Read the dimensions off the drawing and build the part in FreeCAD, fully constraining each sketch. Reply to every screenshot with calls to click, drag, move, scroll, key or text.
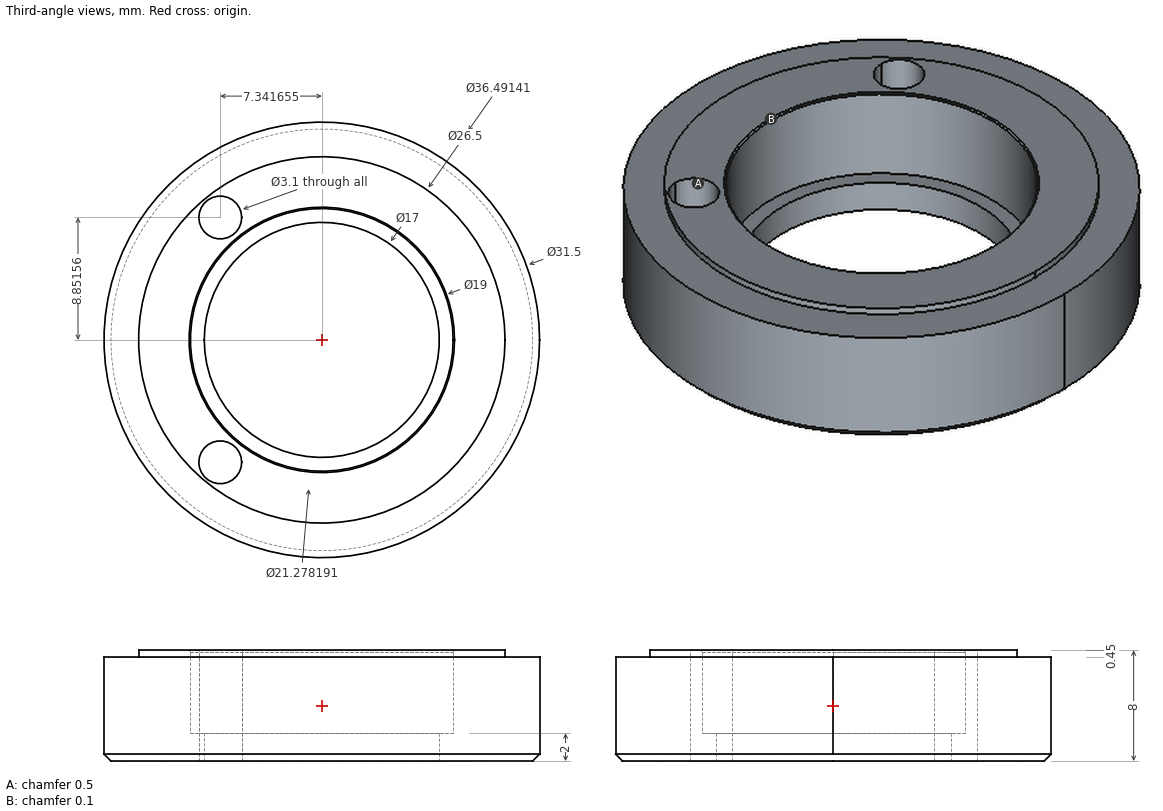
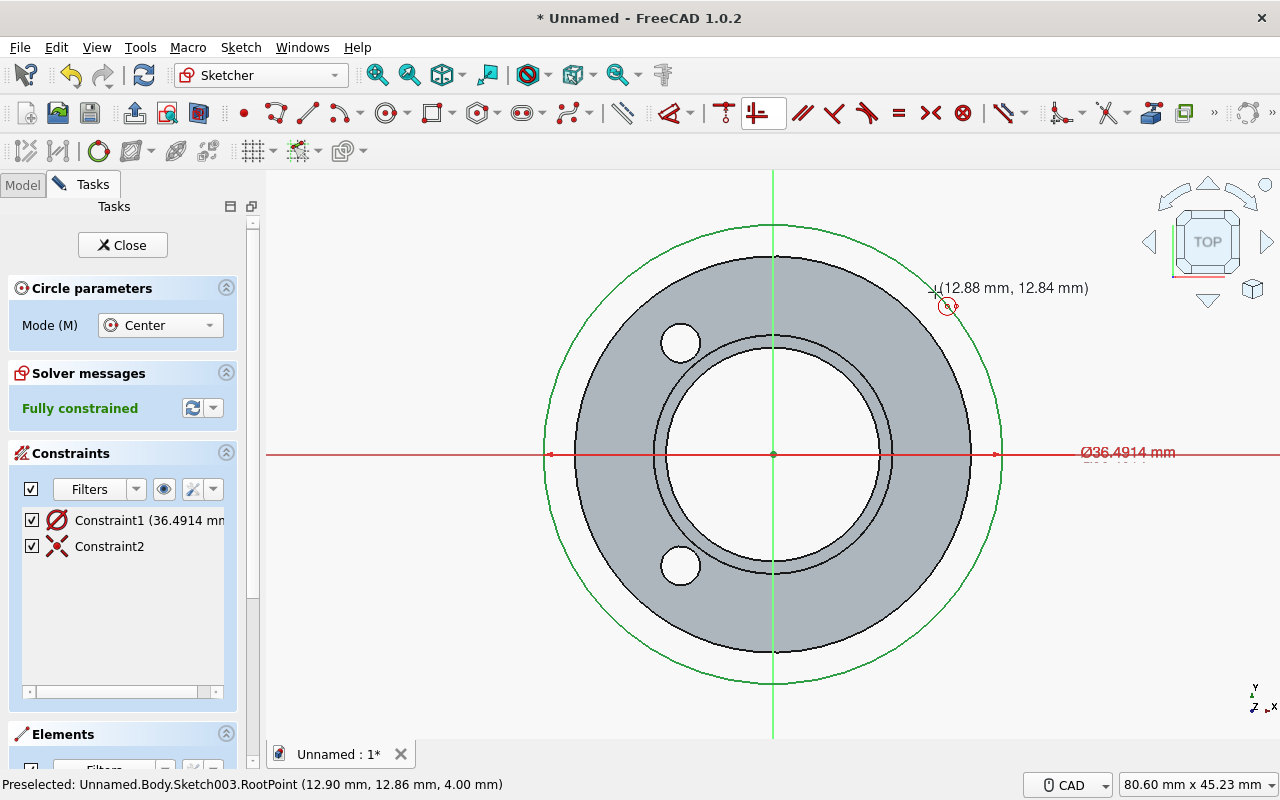
click(773, 454)
move(891, 337)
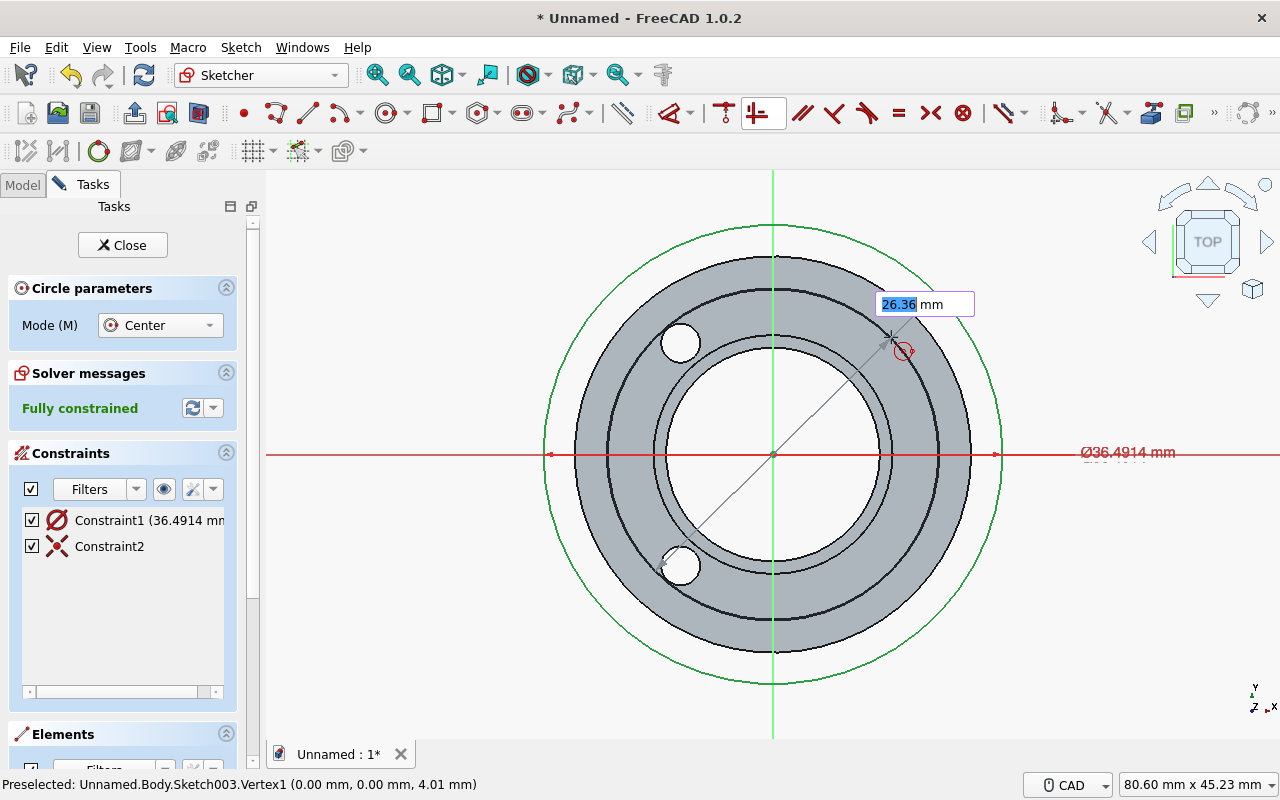
text(26.5)
key(Return)
key(Escape)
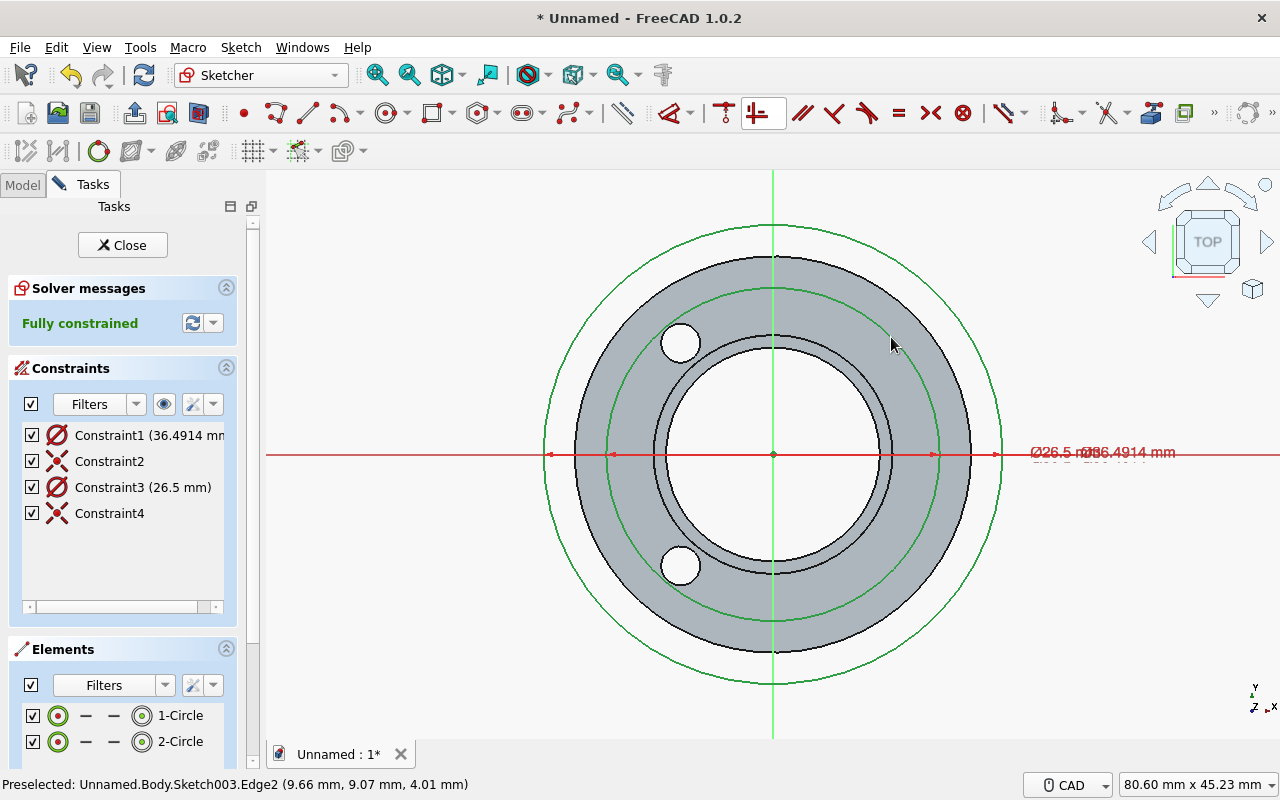
click(123, 245)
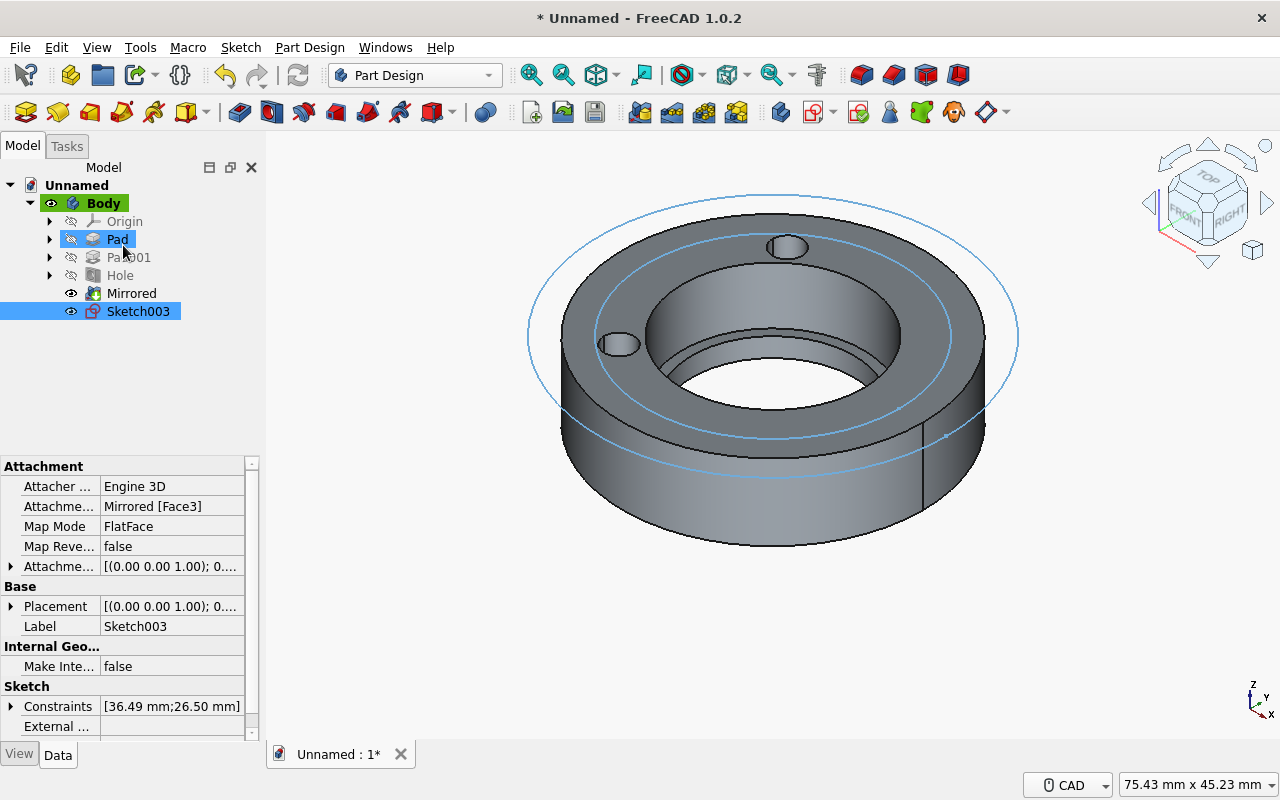
click(240, 112)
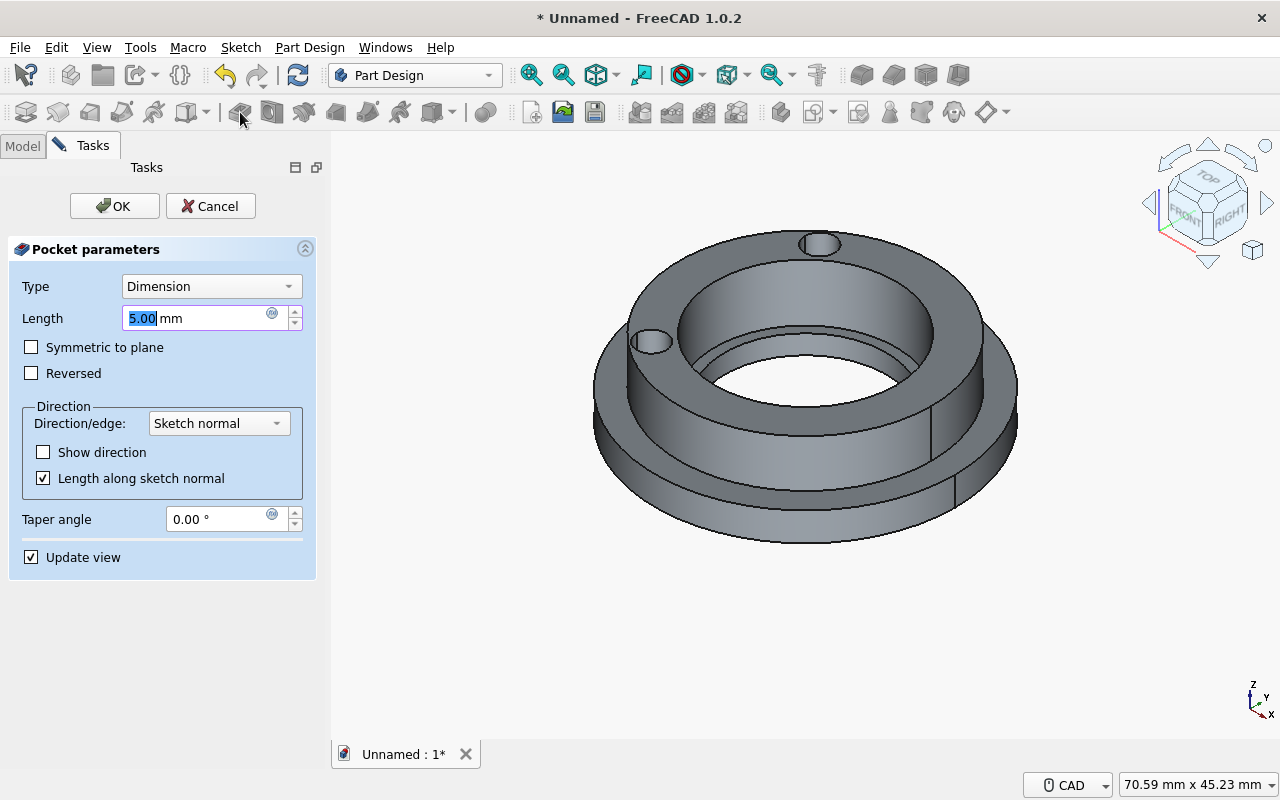
text(0.45)
key(Tab)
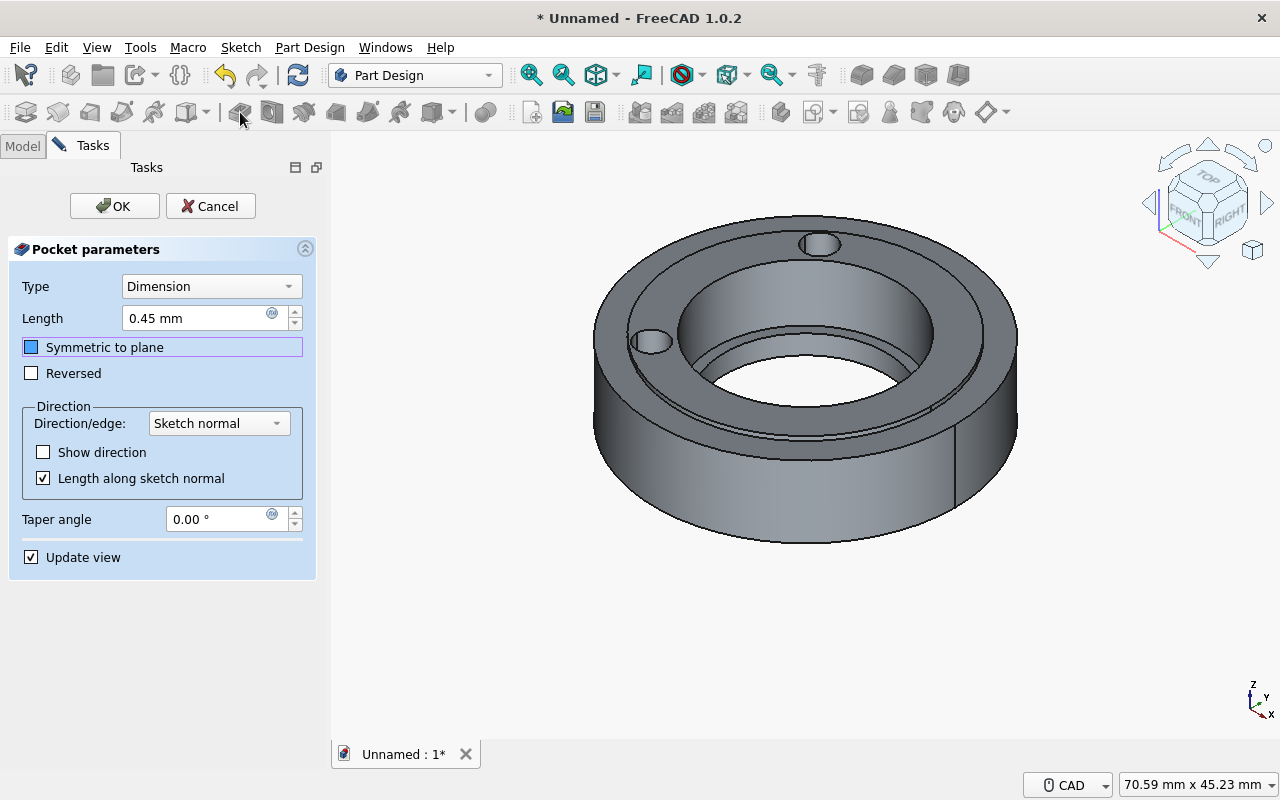
click(115, 206)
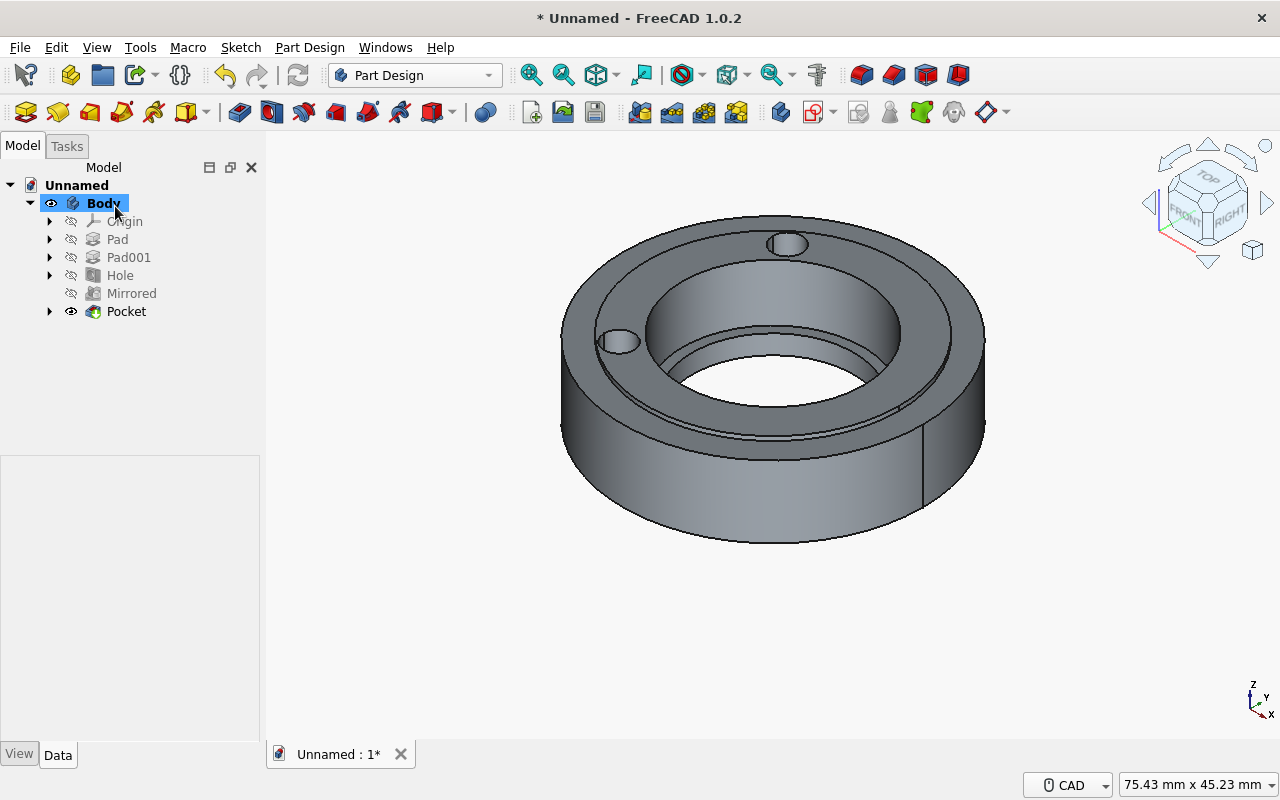
key(2)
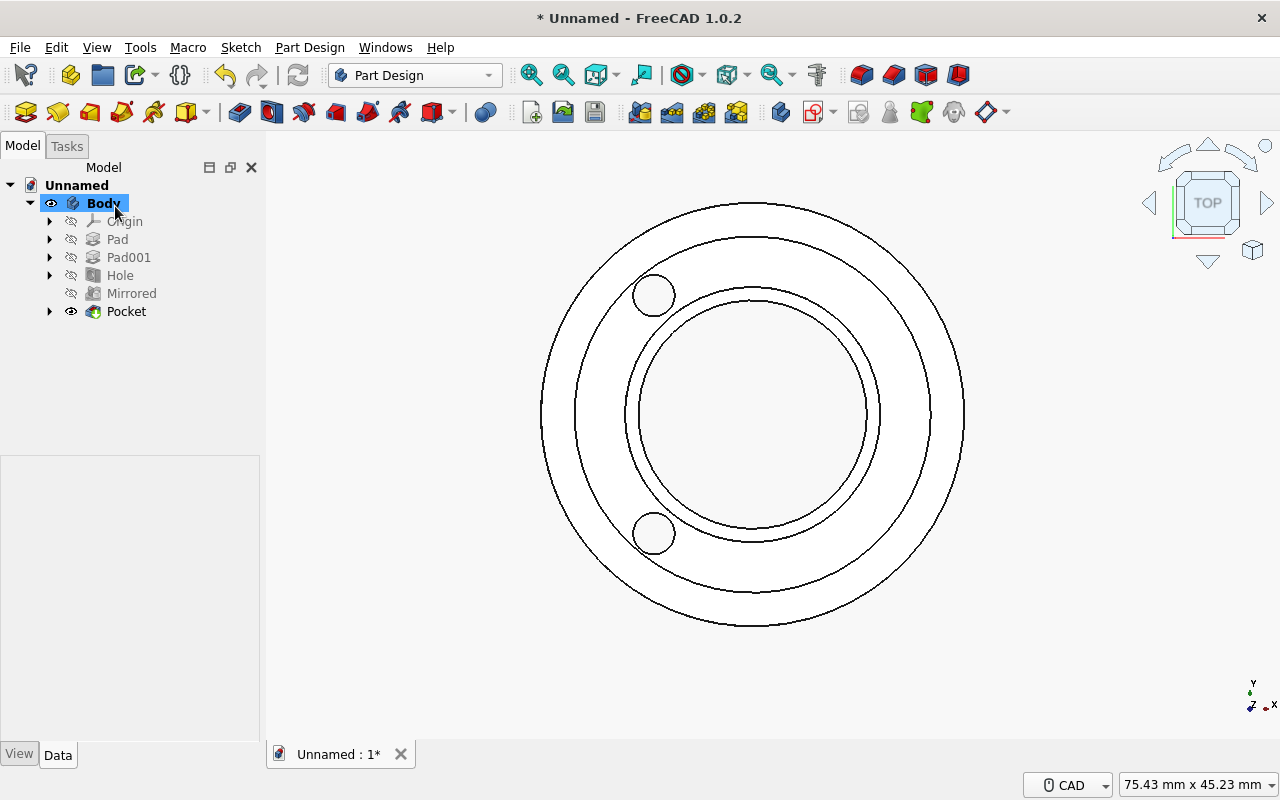
key(0)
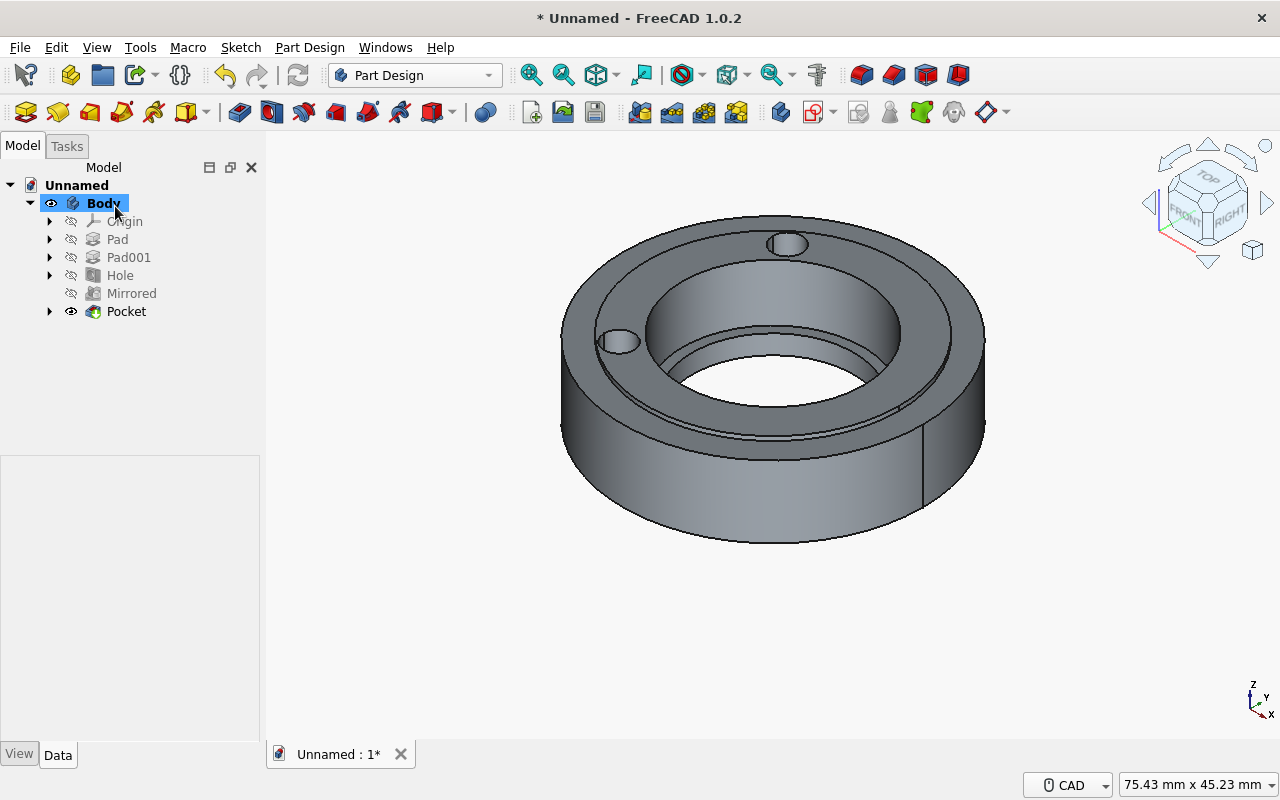
key(1)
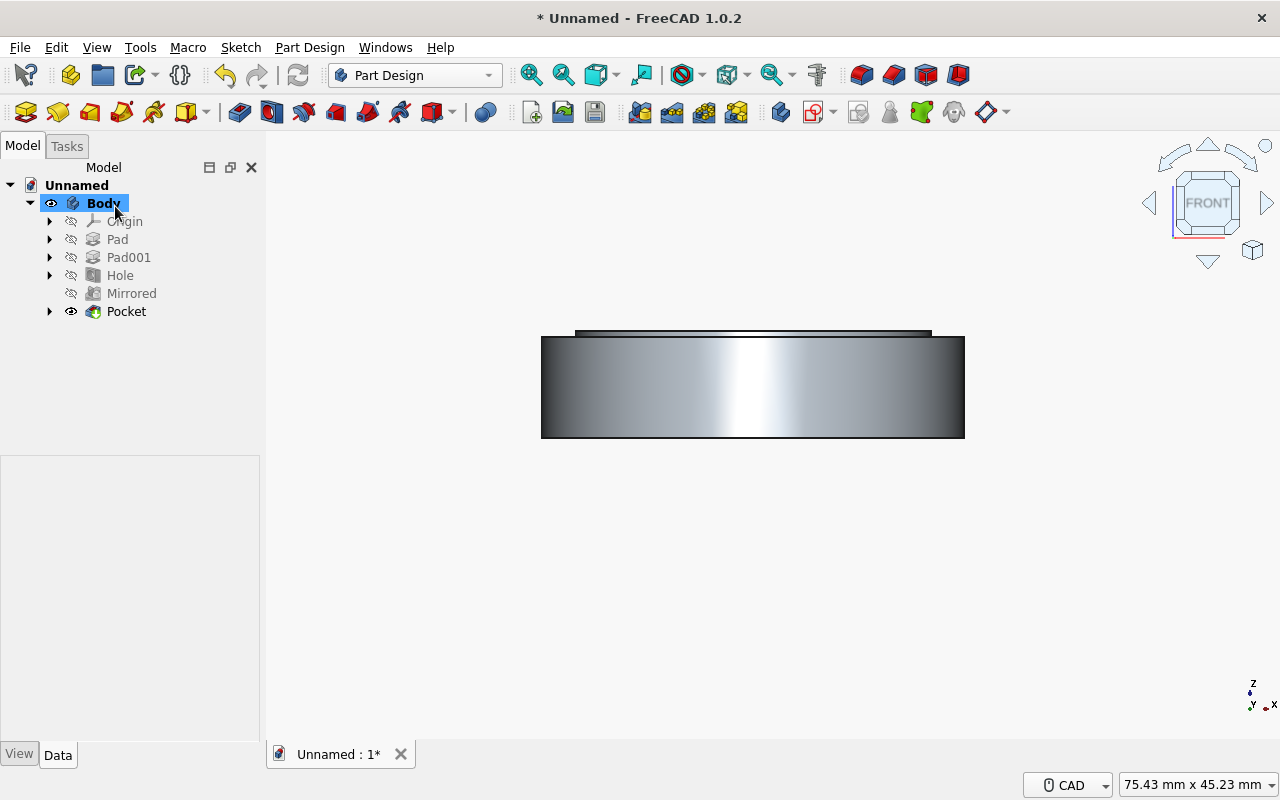
click(532, 76)